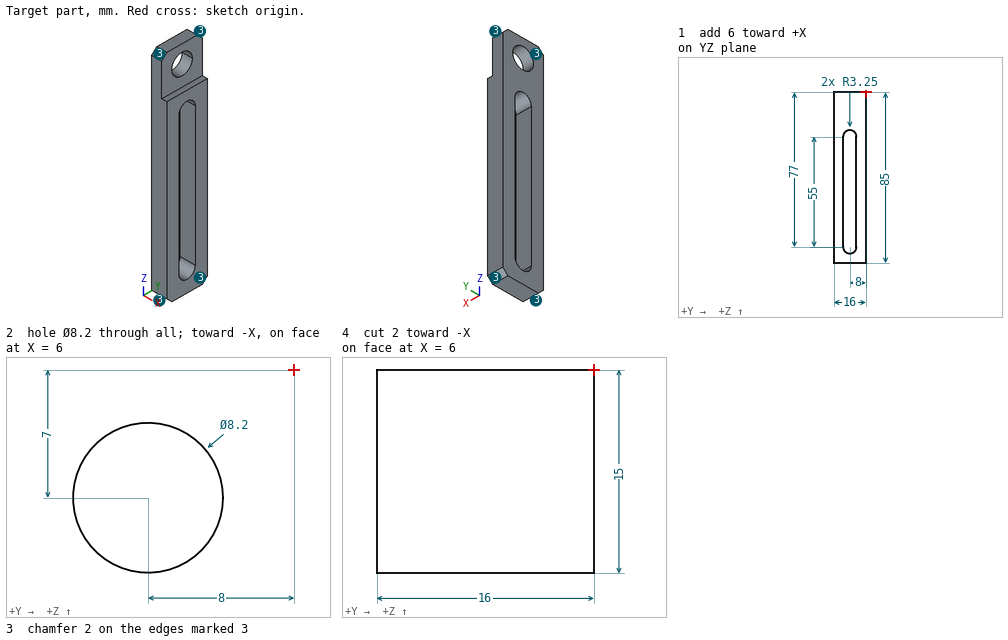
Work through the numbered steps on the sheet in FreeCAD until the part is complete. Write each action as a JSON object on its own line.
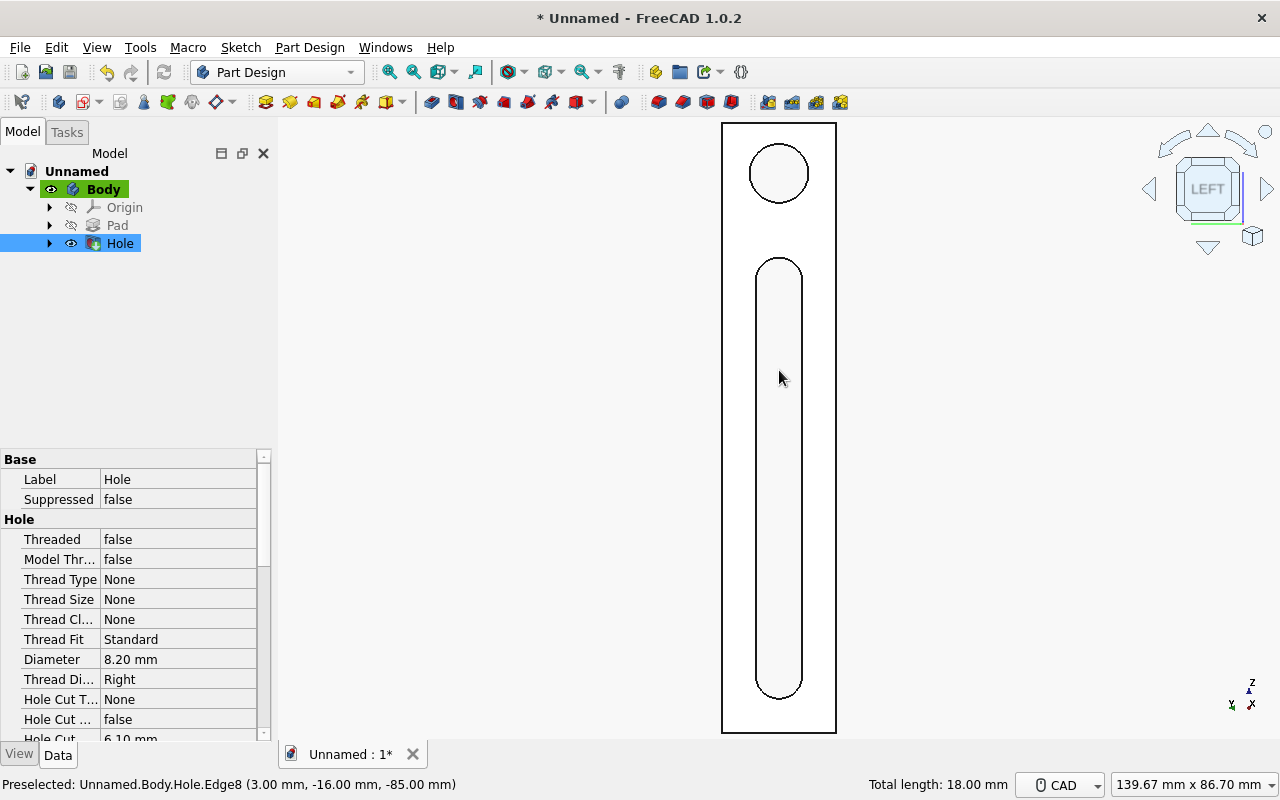
{"action": "key", "text": "v 3"}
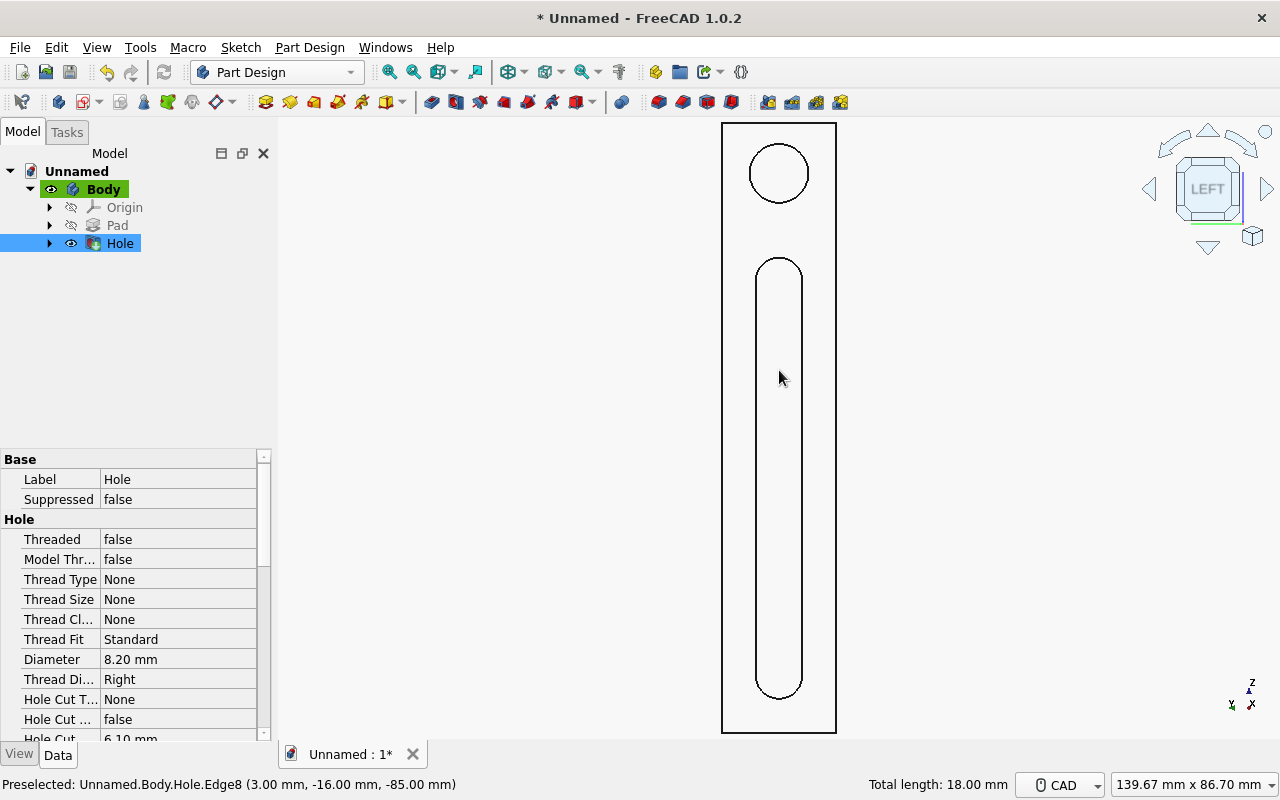
{"action": "key", "text": "0"}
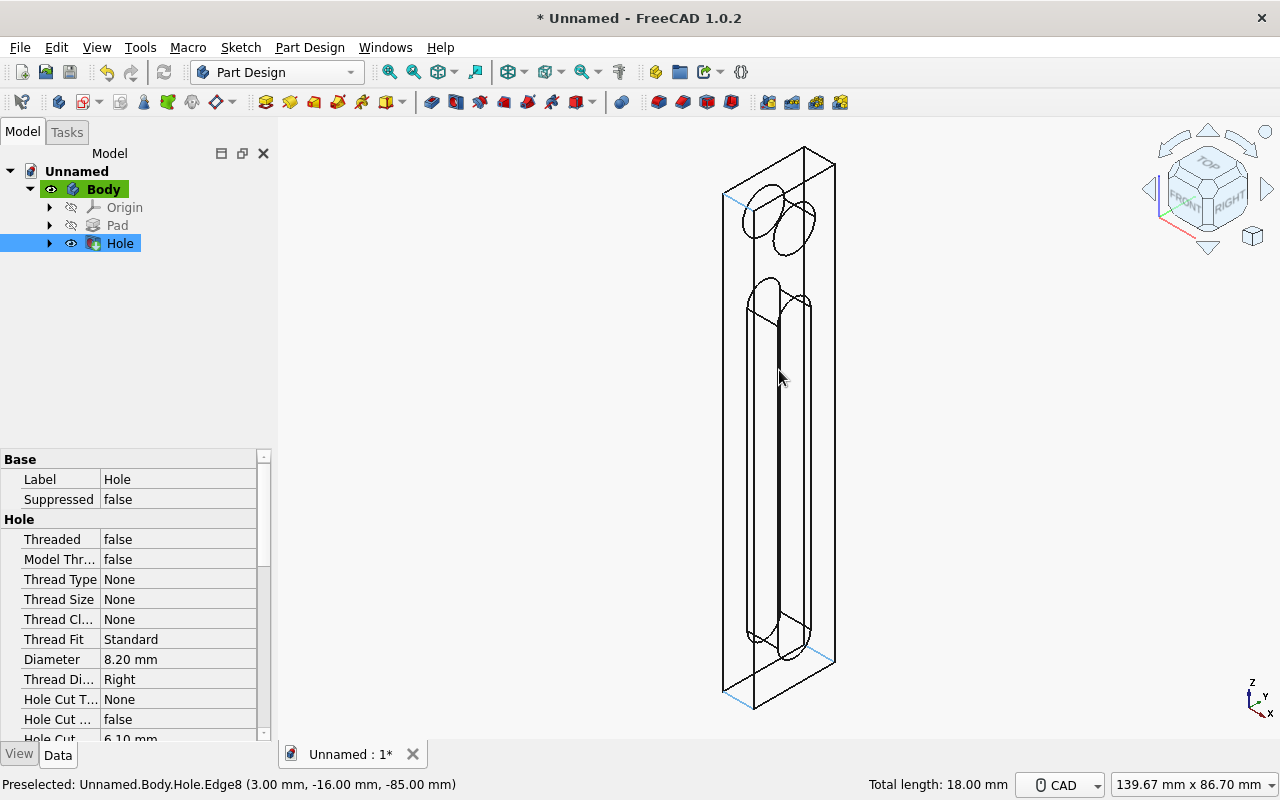
{"action": "left_click", "coordinate": [820, 155], "text": "ctrl"}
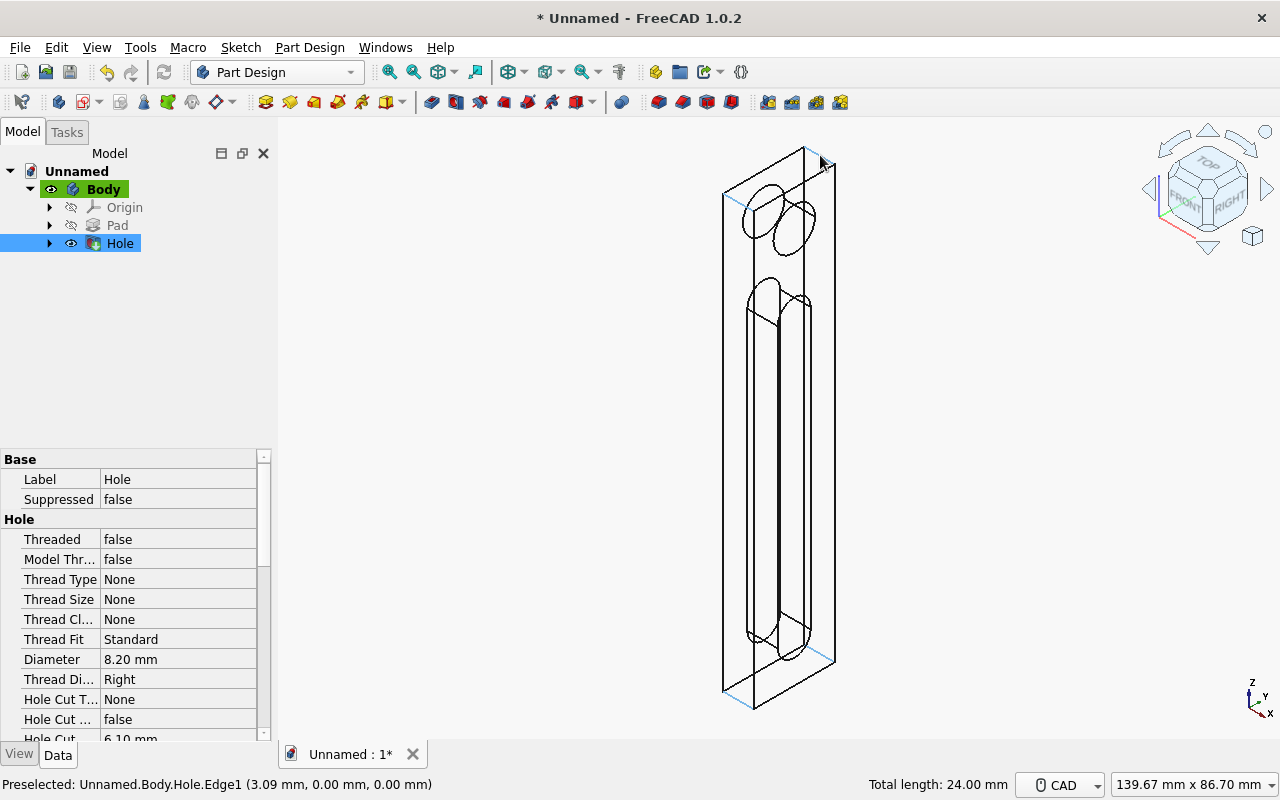
{"action": "key", "text": "v 1"}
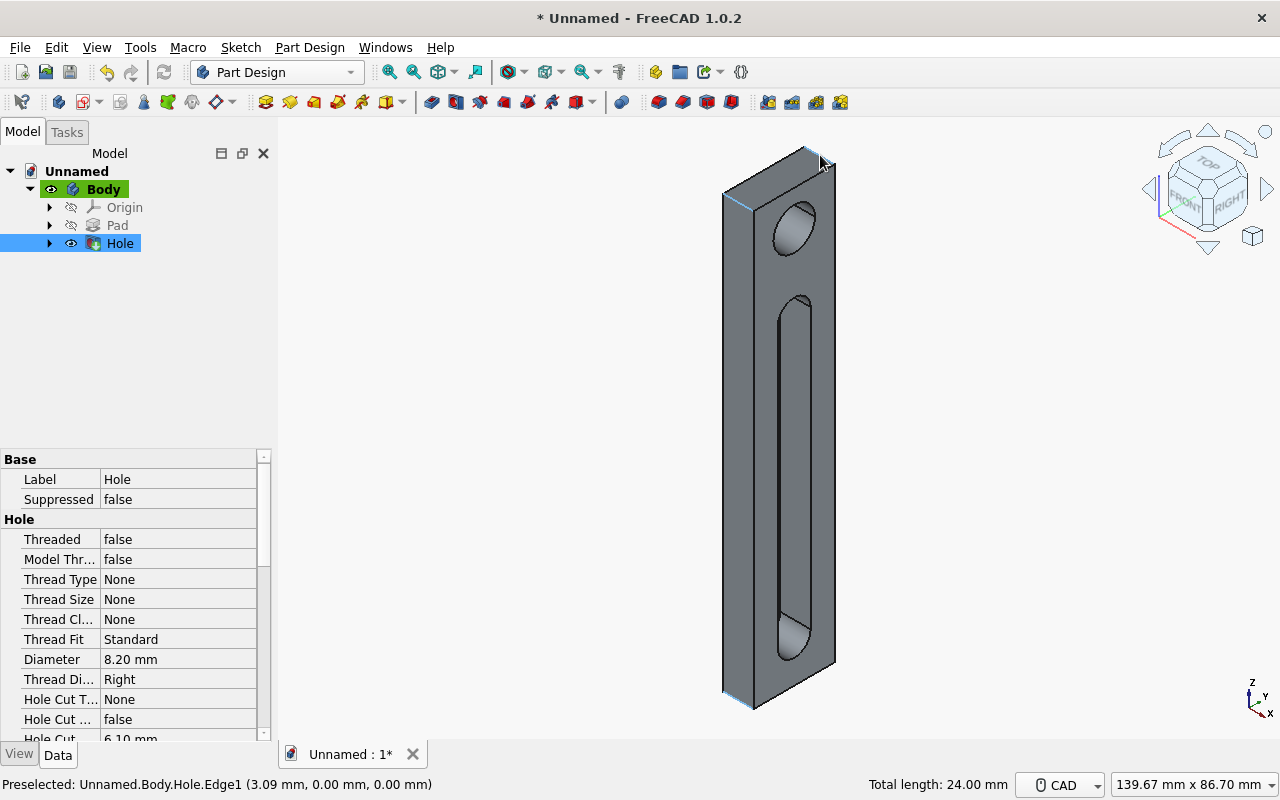
{"action": "left_click", "coordinate": [684, 102]}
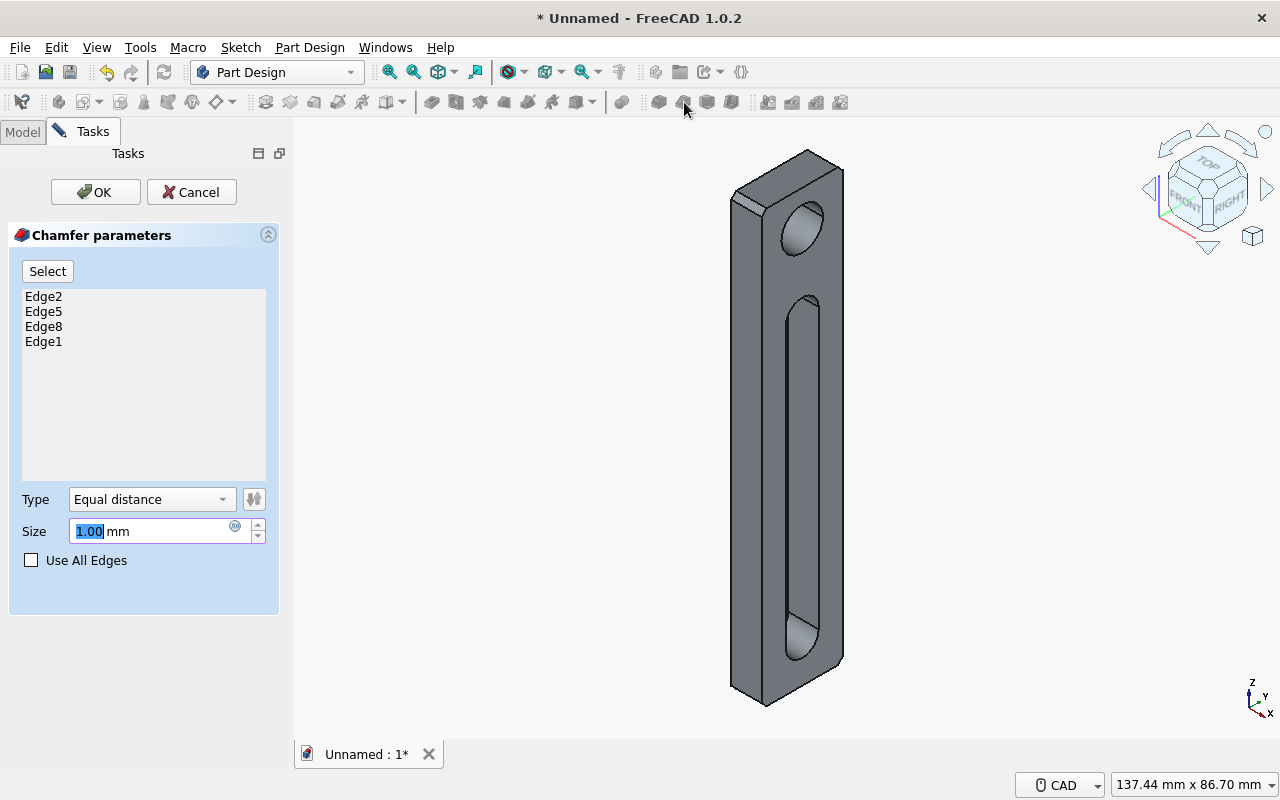
{"action": "type", "text": "2"}
{"action": "key", "text": "Tab"}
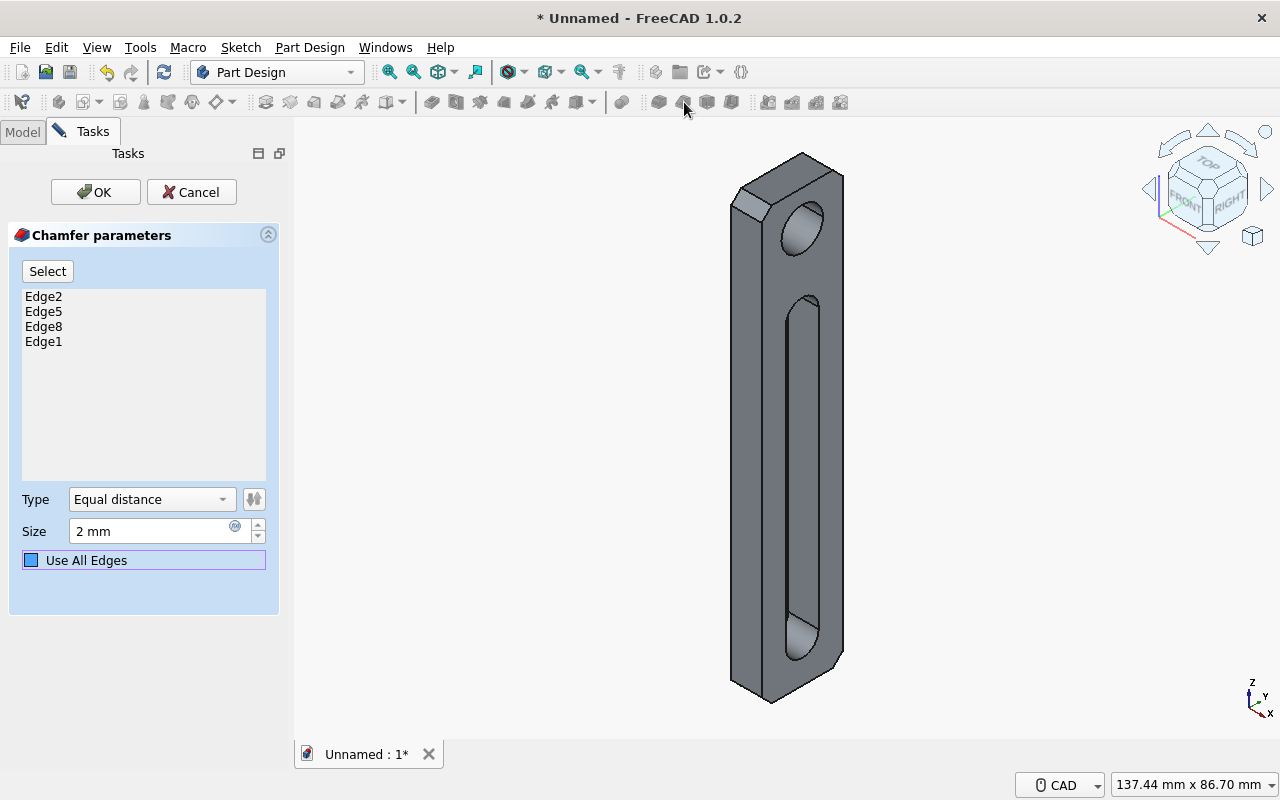
{"action": "left_click", "coordinate": [96, 192]}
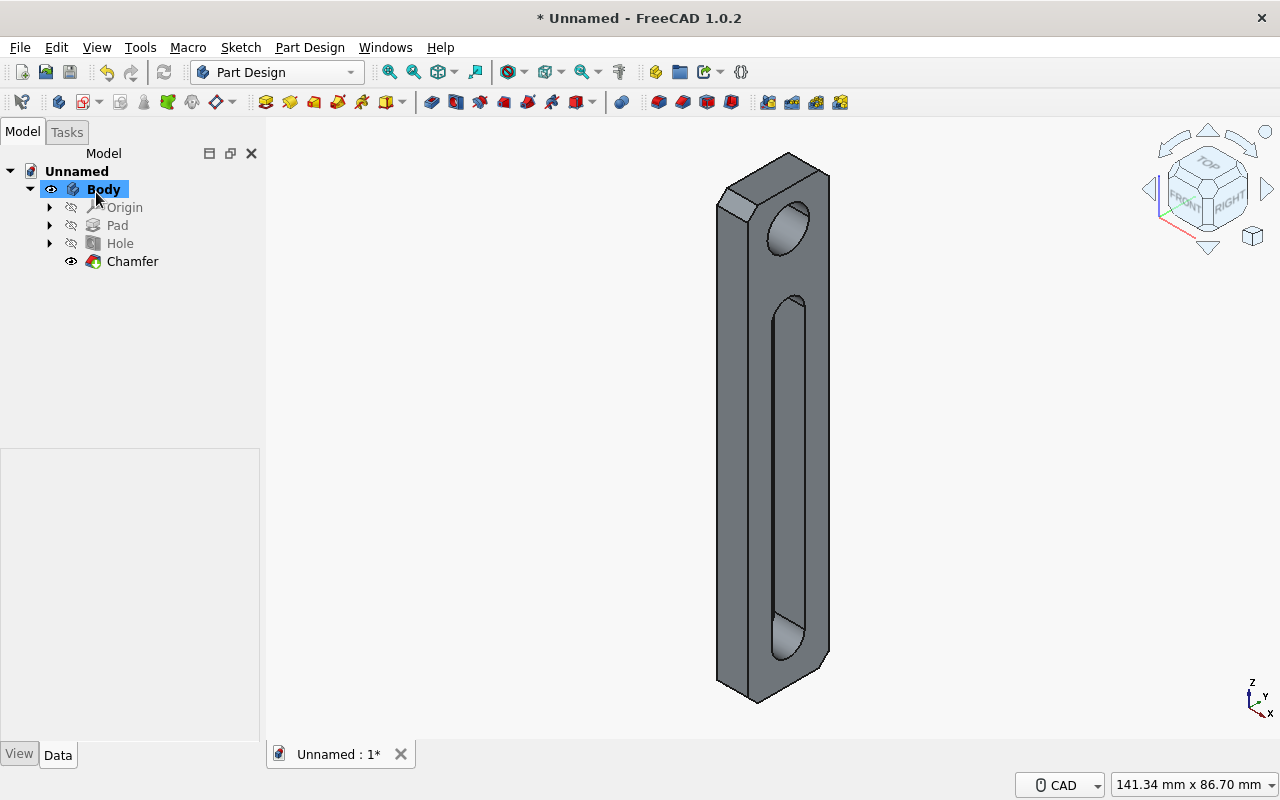
{"action": "left_click", "coordinate": [811, 280]}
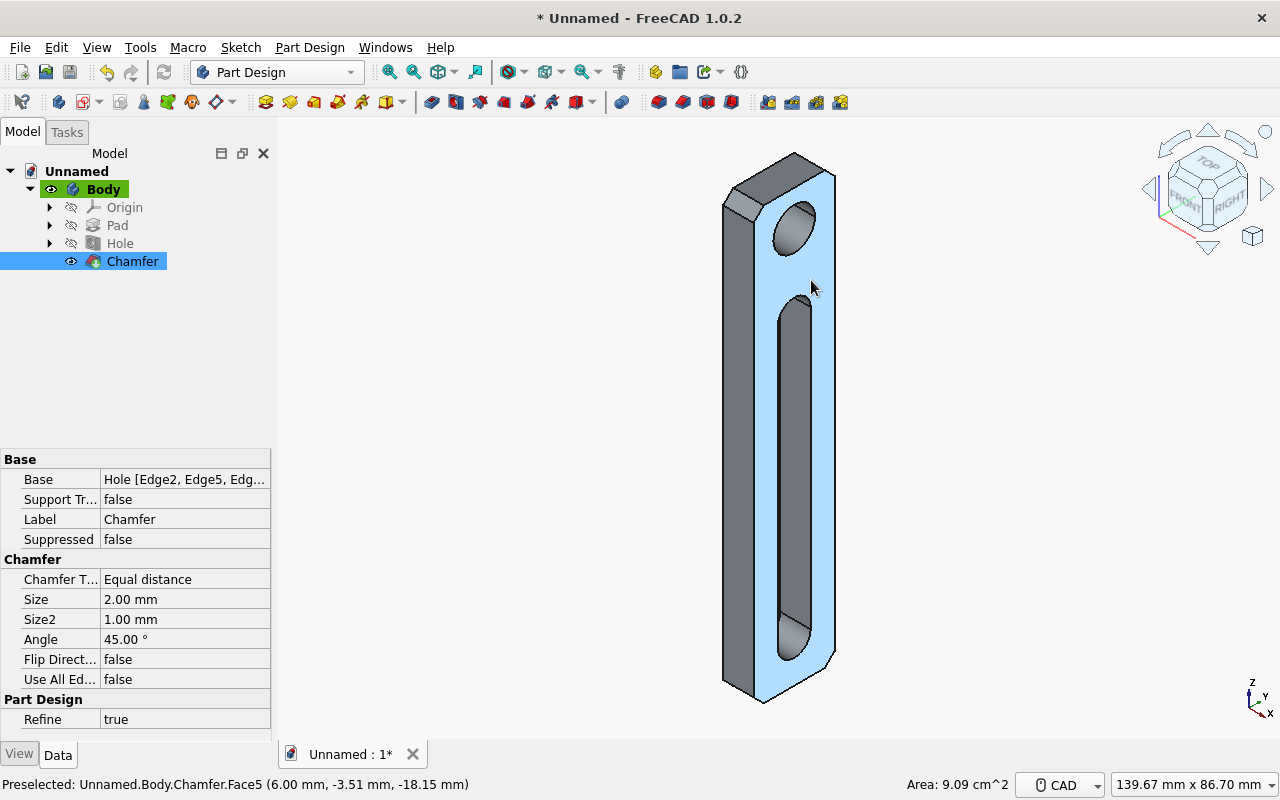
{"action": "left_click", "coordinate": [84, 102]}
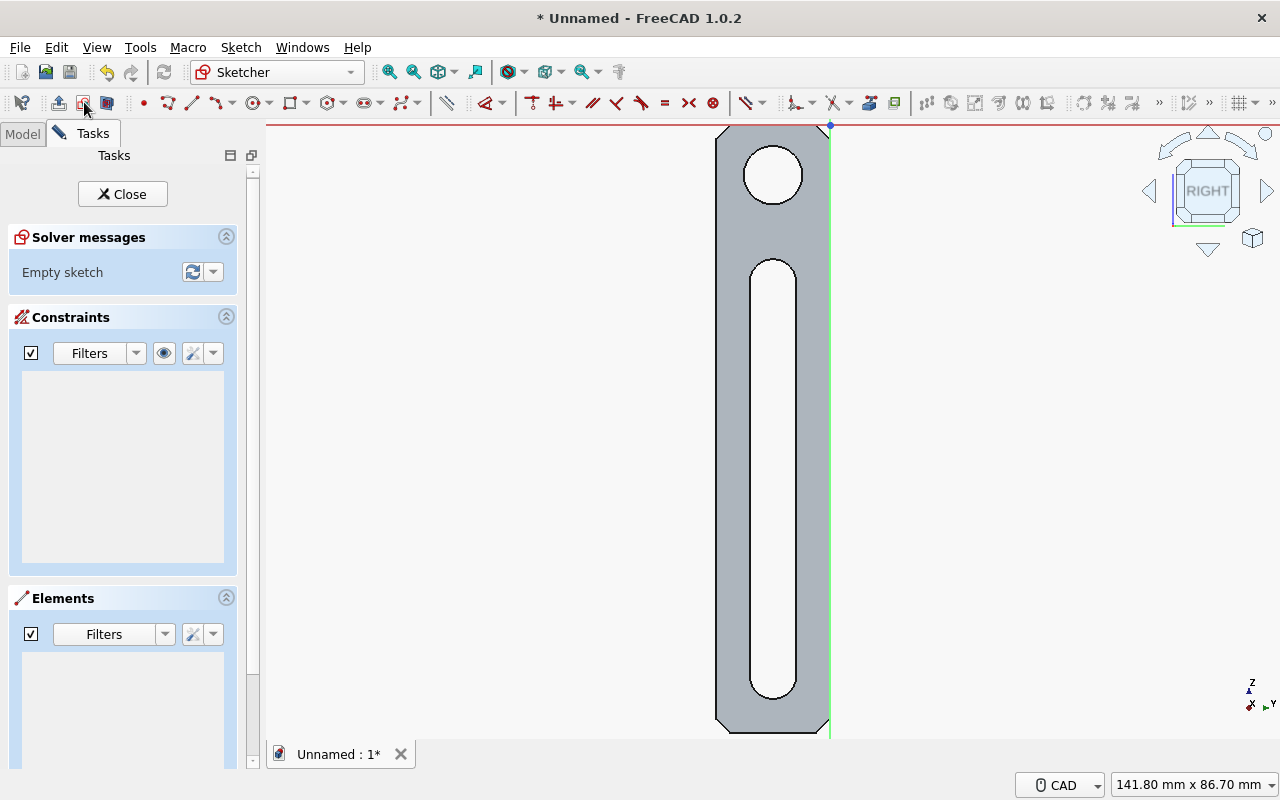
{"action": "scroll", "coordinate": [704, 429], "scroll_direction": "down", "scroll_amount": 5}